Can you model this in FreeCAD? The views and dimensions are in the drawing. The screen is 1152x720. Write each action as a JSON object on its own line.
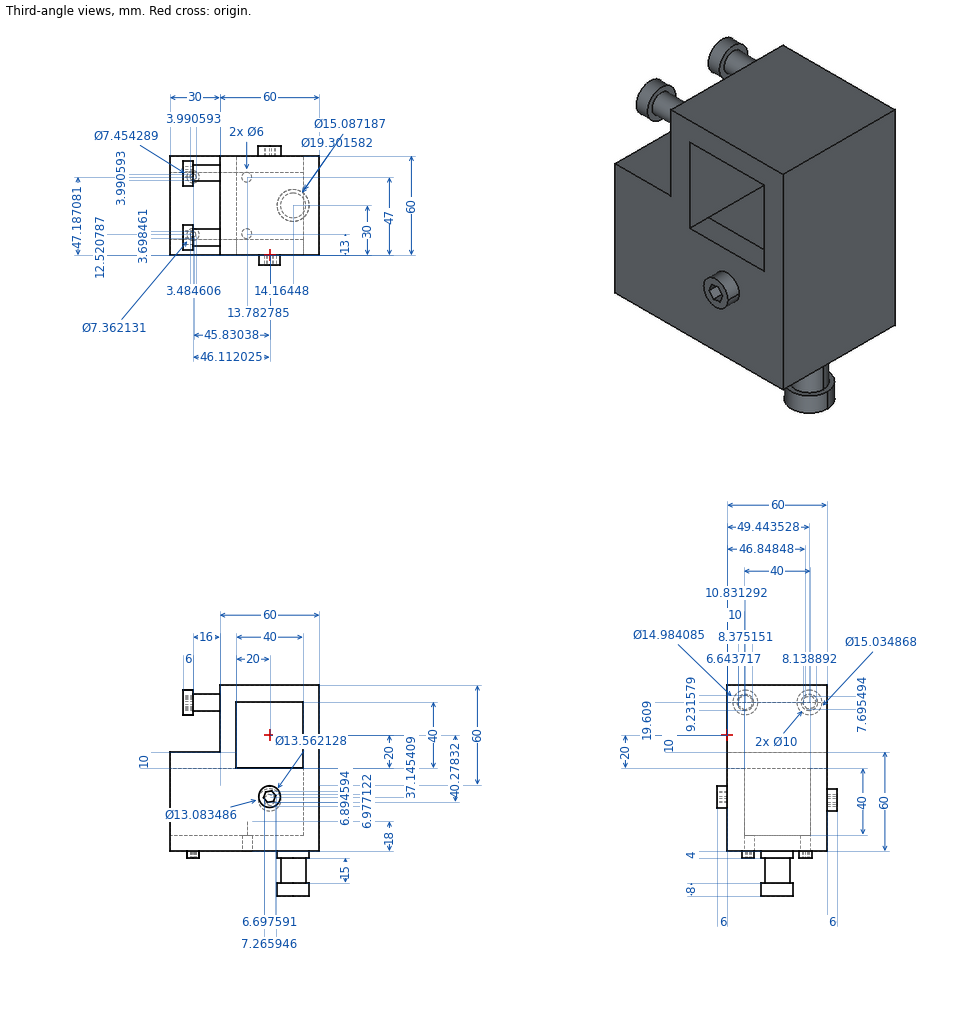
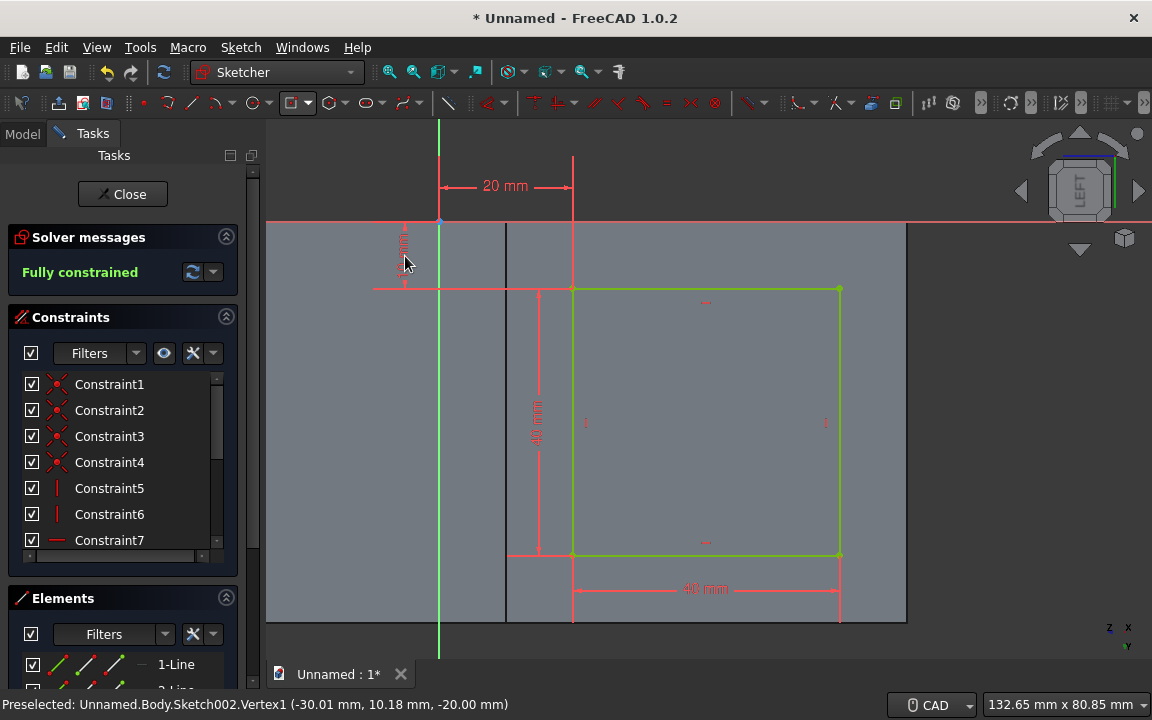
{"action": "left_click", "coordinate": [123, 194]}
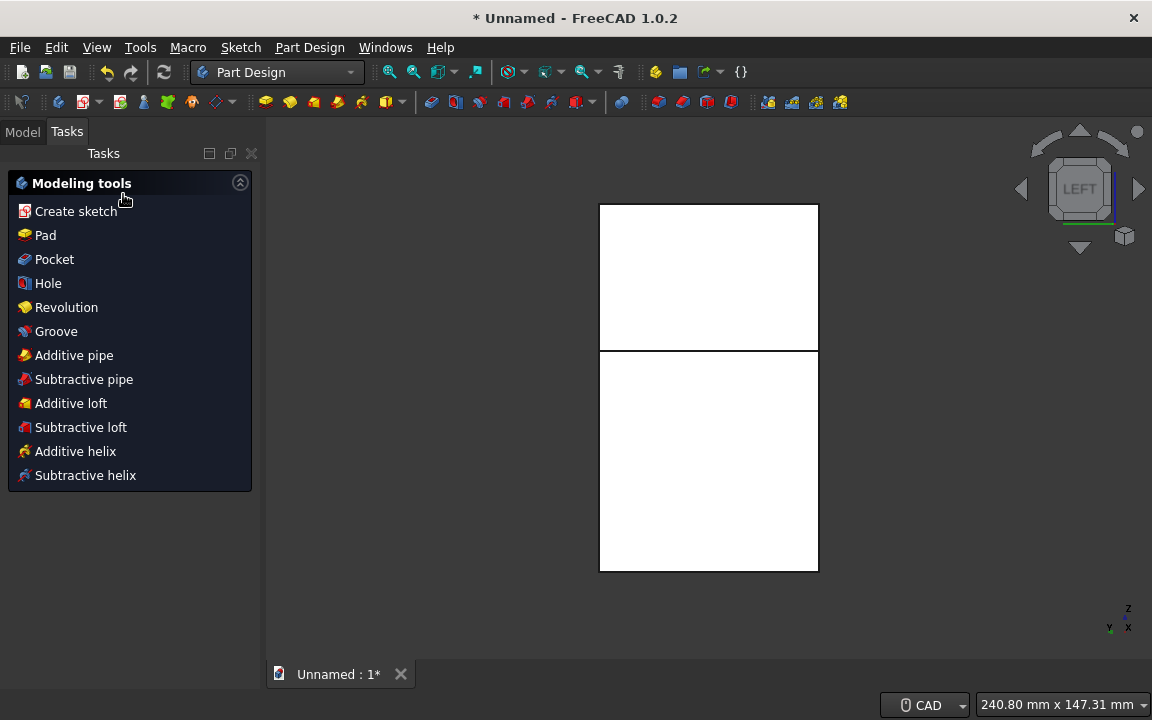
{"action": "left_click", "coordinate": [432, 102]}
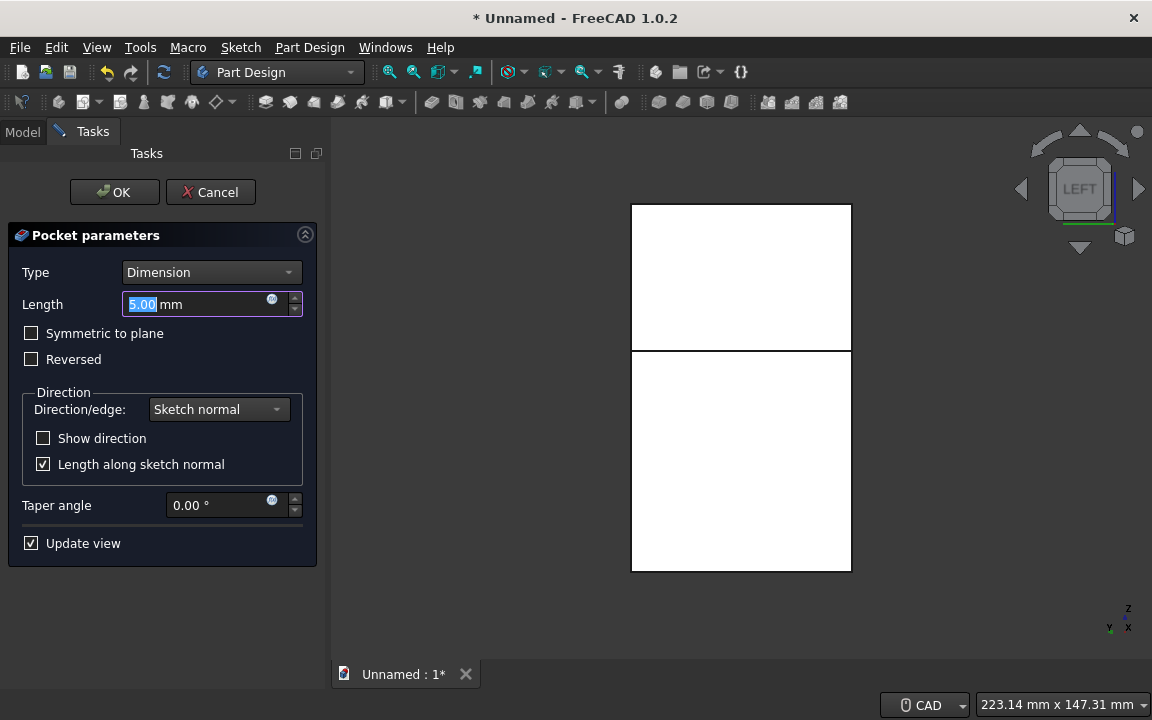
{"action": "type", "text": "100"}
{"action": "key", "text": "Tab"}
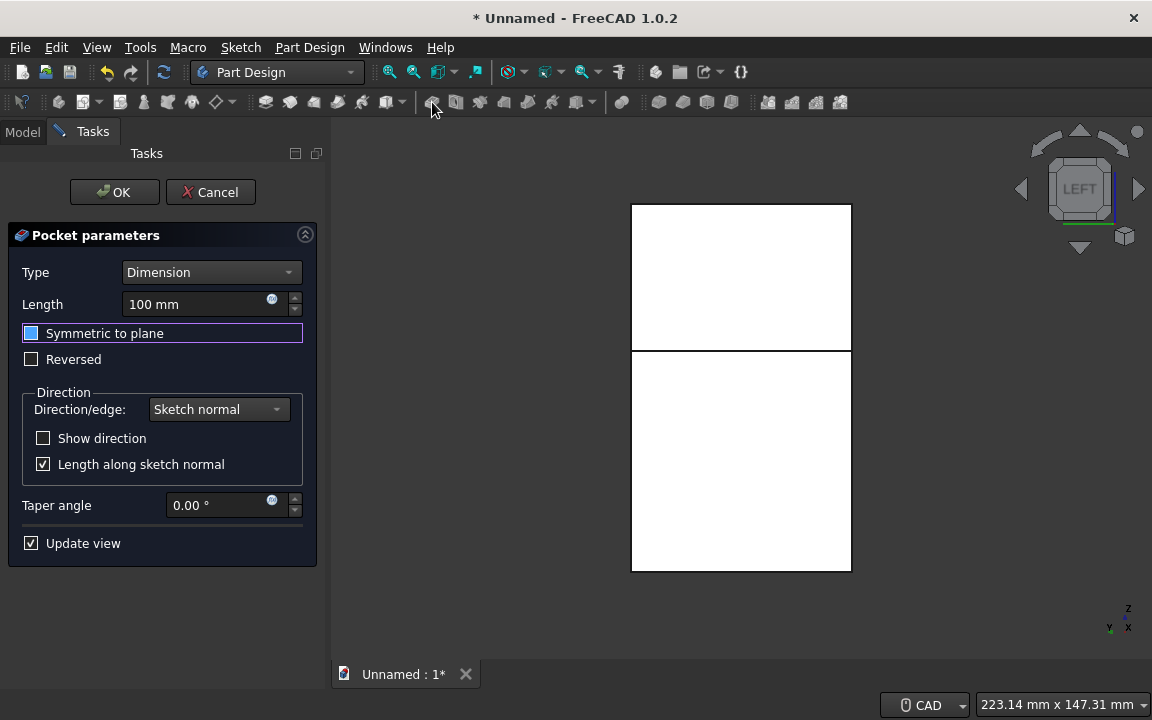
{"action": "left_click", "coordinate": [30, 333]}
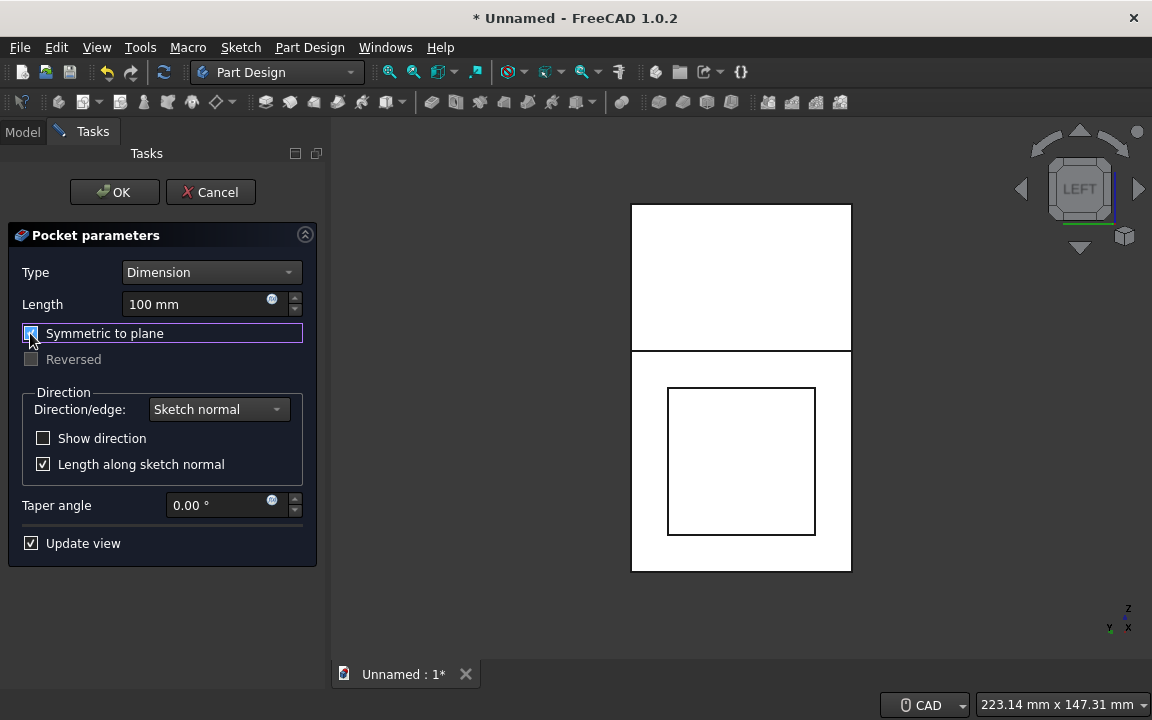
{"action": "left_click", "coordinate": [115, 192]}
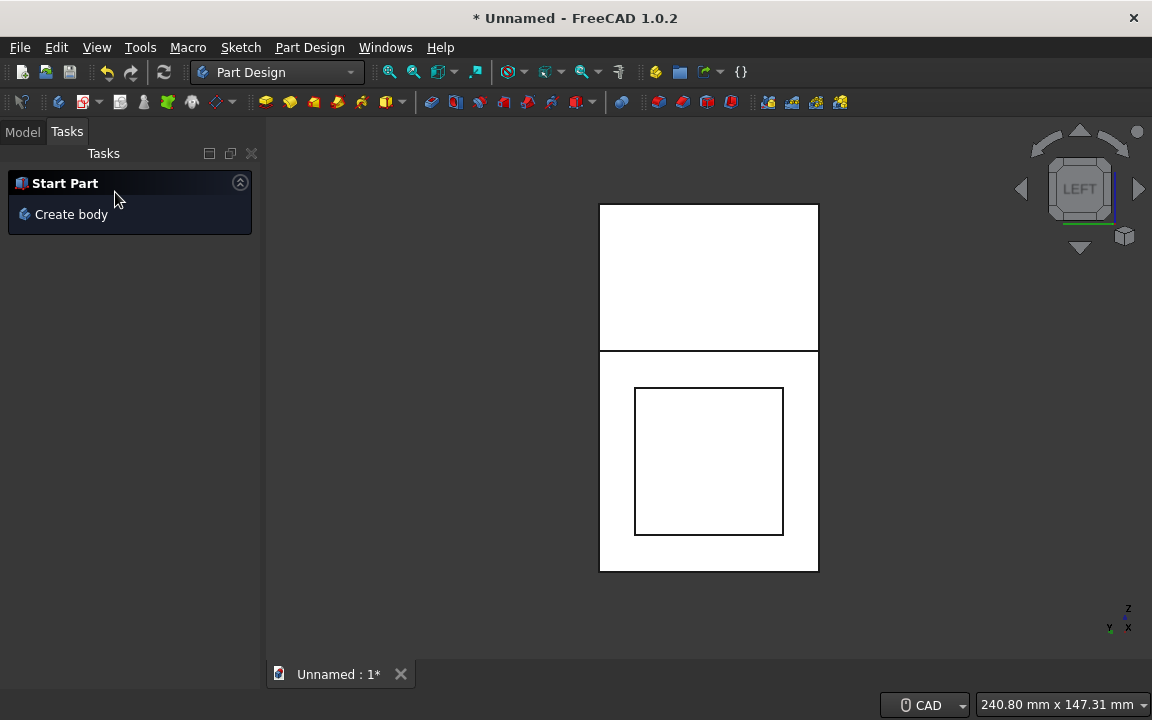
{"action": "key", "text": "4"}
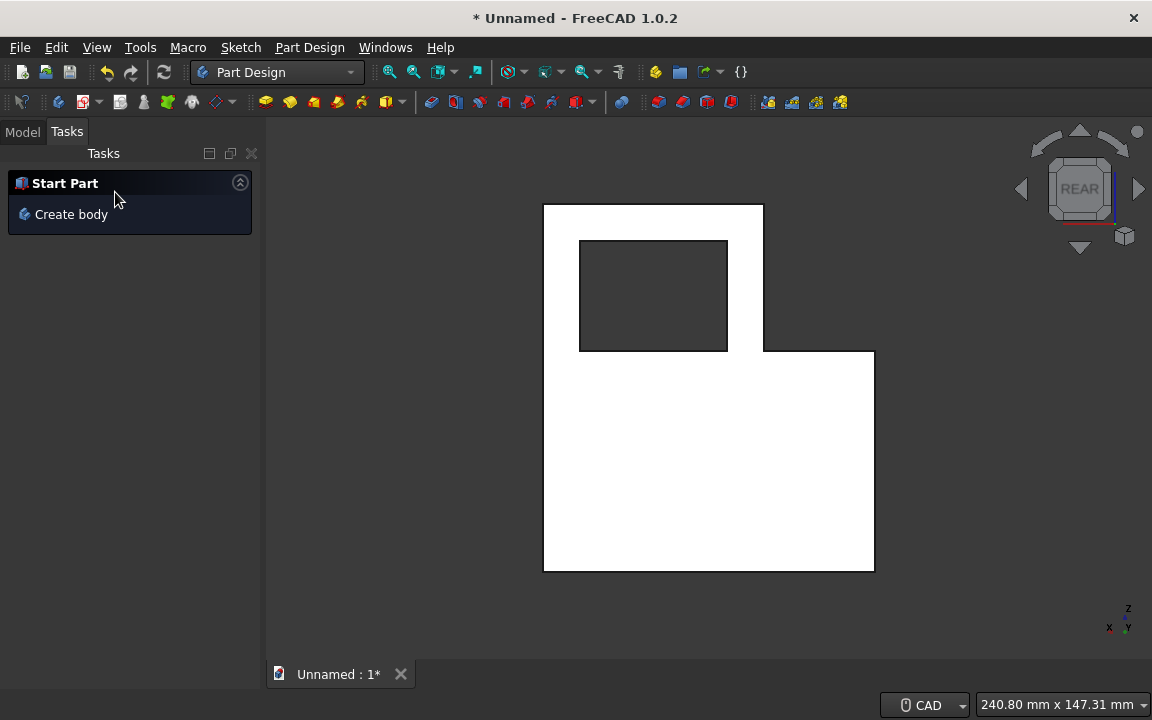
{"action": "left_click", "coordinate": [756, 440]}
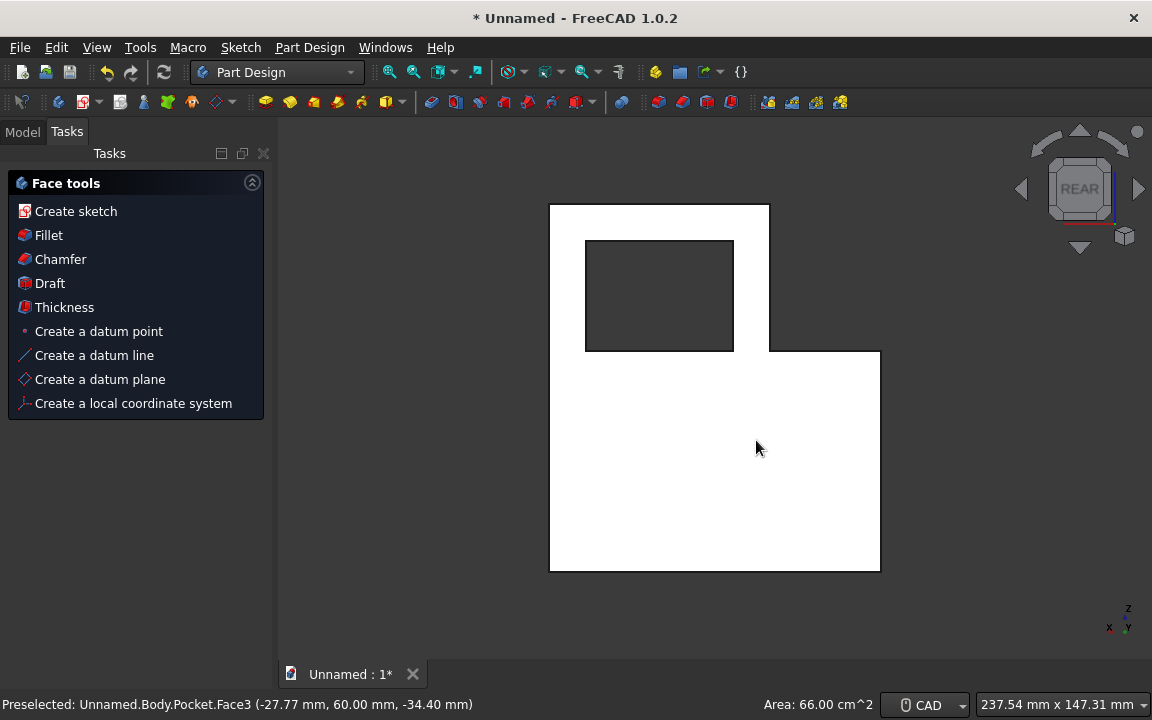
{"action": "left_click", "coordinate": [84, 102]}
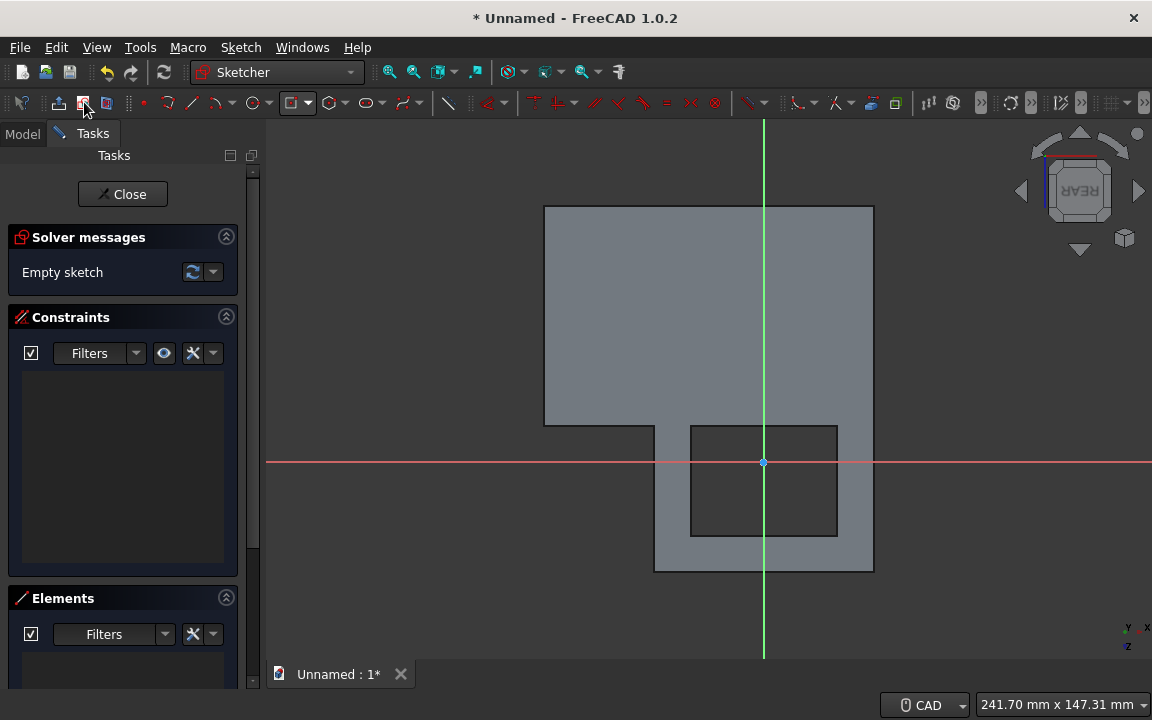
{"action": "scroll", "coordinate": [817, 441], "scroll_direction": "up", "scroll_amount": 6}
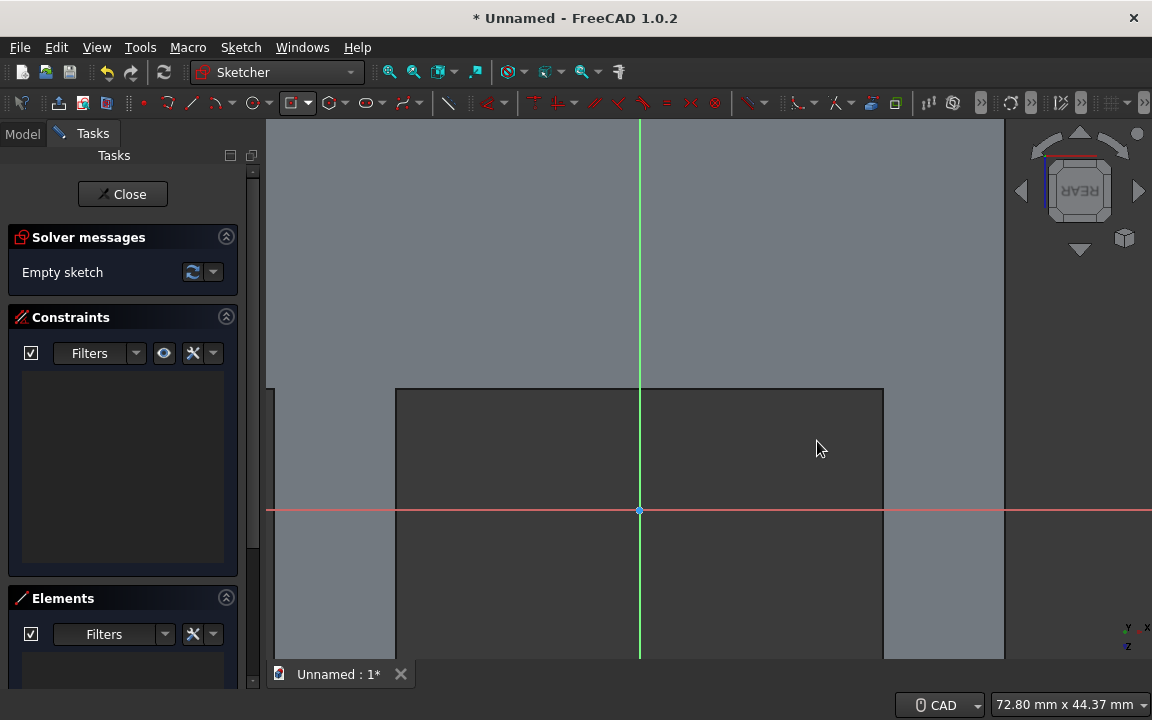
{"action": "key", "text": "g r"}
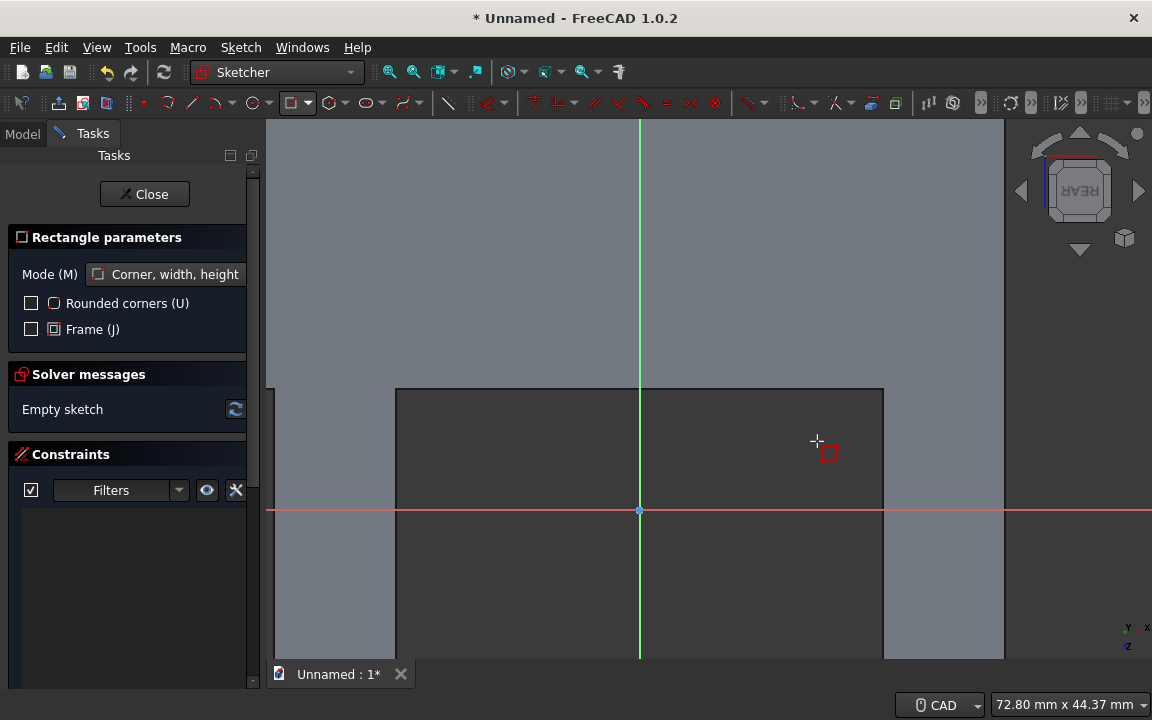
{"action": "left_click", "coordinate": [396, 267]}
{"action": "left_click", "coordinate": [883, 389]}
{"action": "key", "text": "Escape"}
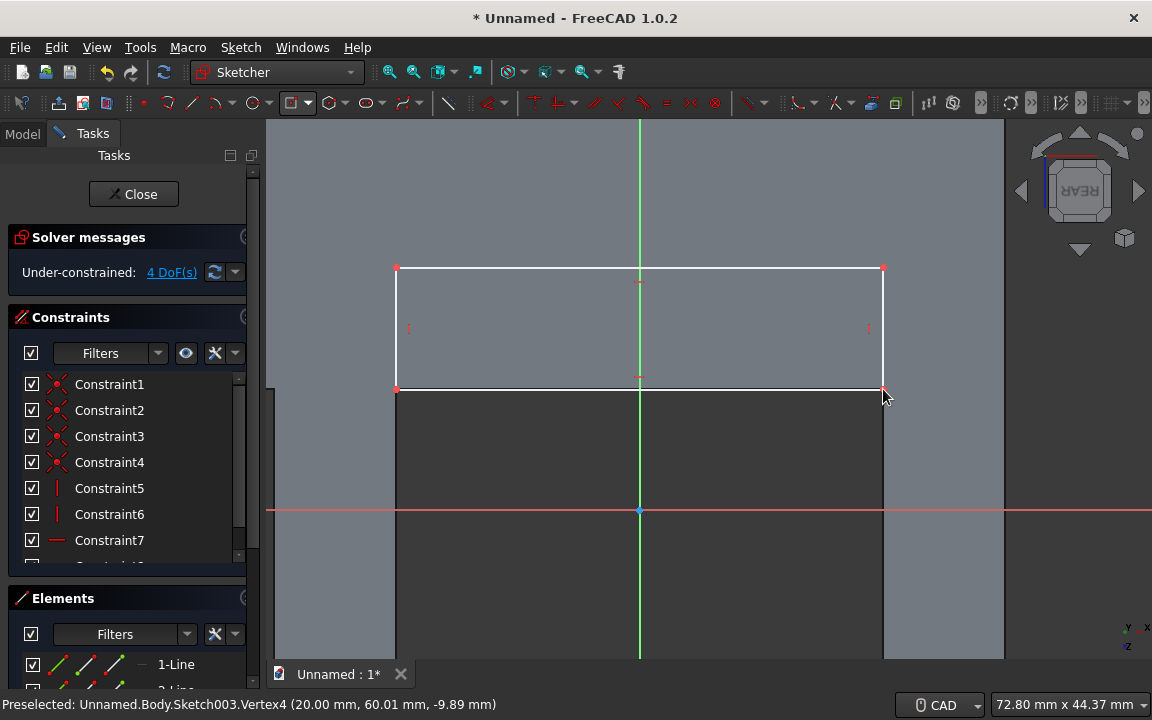
{"action": "left_click", "coordinate": [488, 104]}